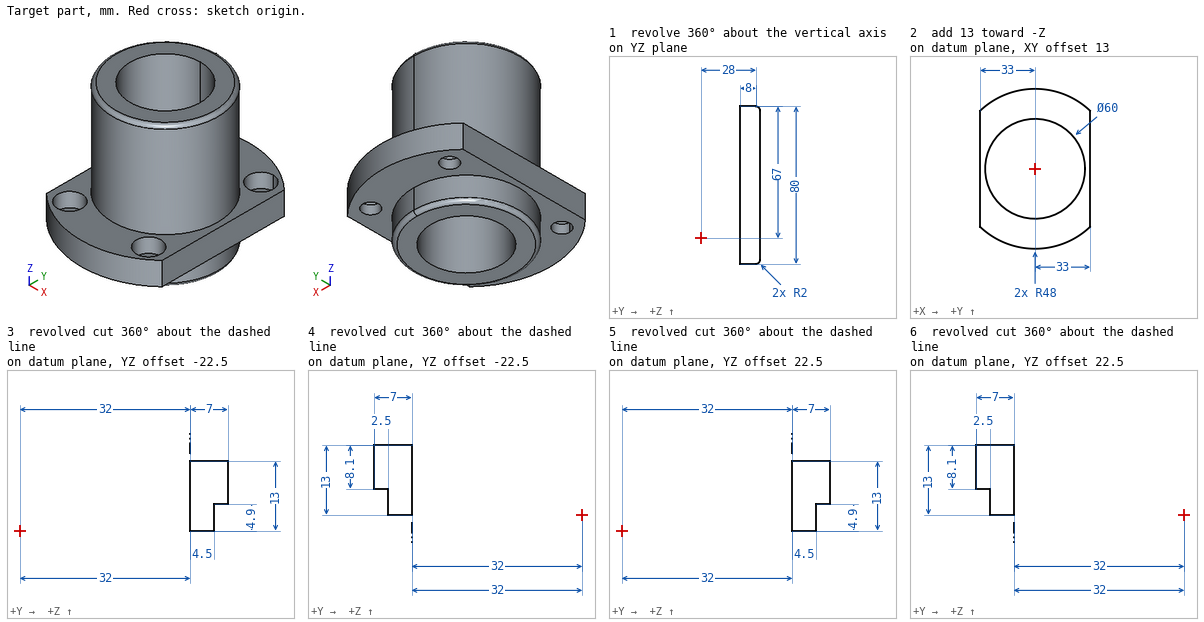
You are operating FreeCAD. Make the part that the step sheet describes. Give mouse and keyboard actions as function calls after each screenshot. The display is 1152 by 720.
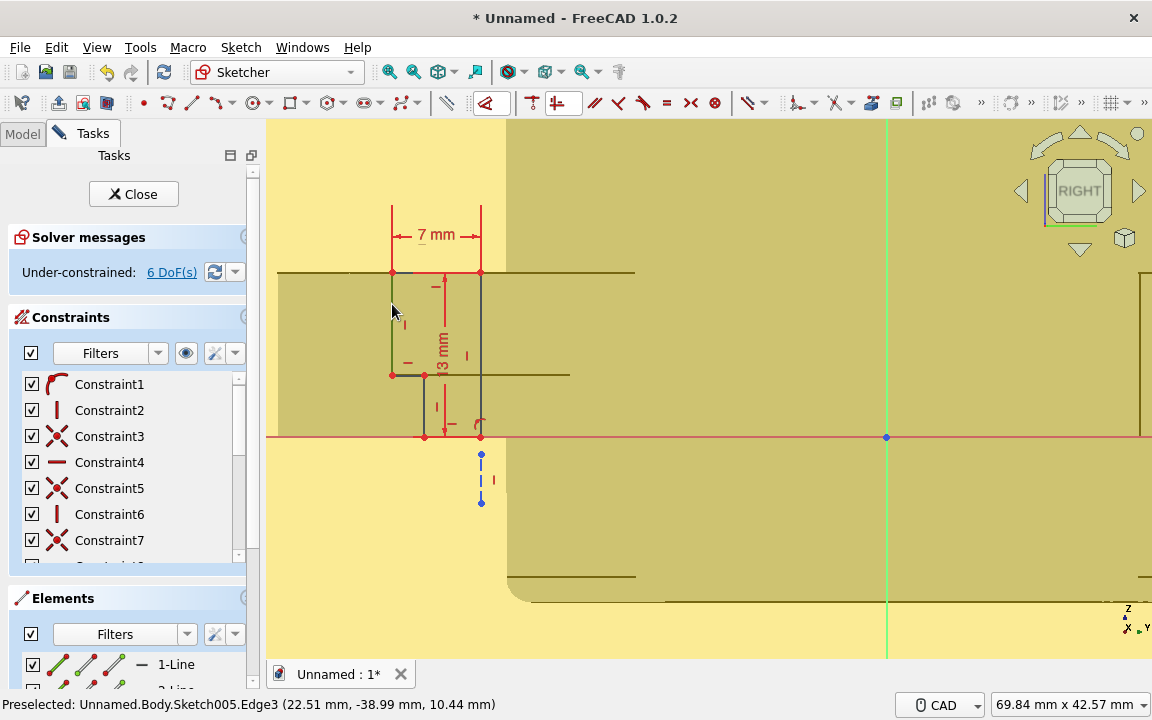
click(504, 104)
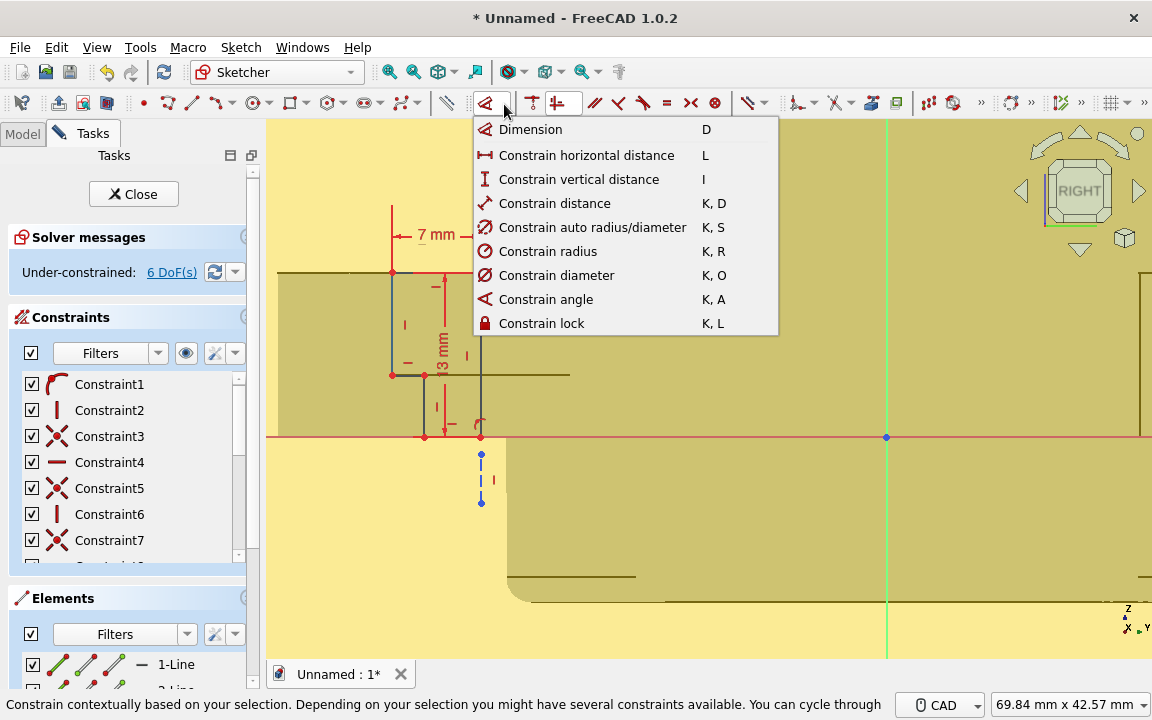
click(626, 179)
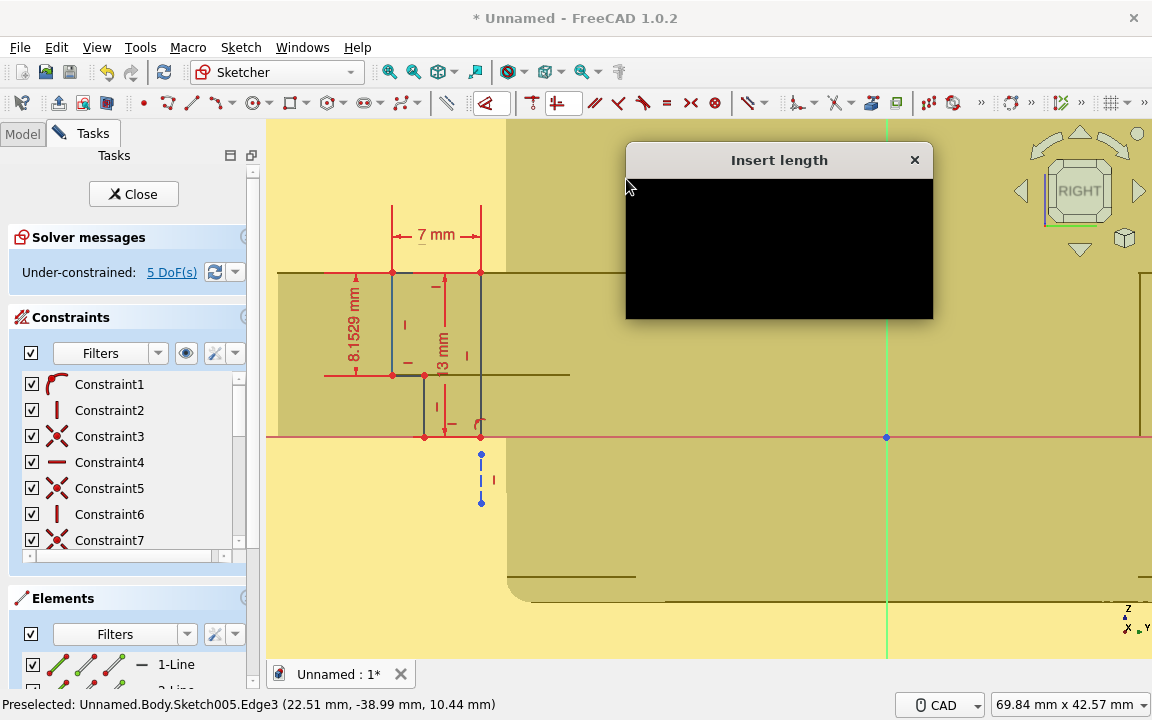
text(8.1)
key(Return)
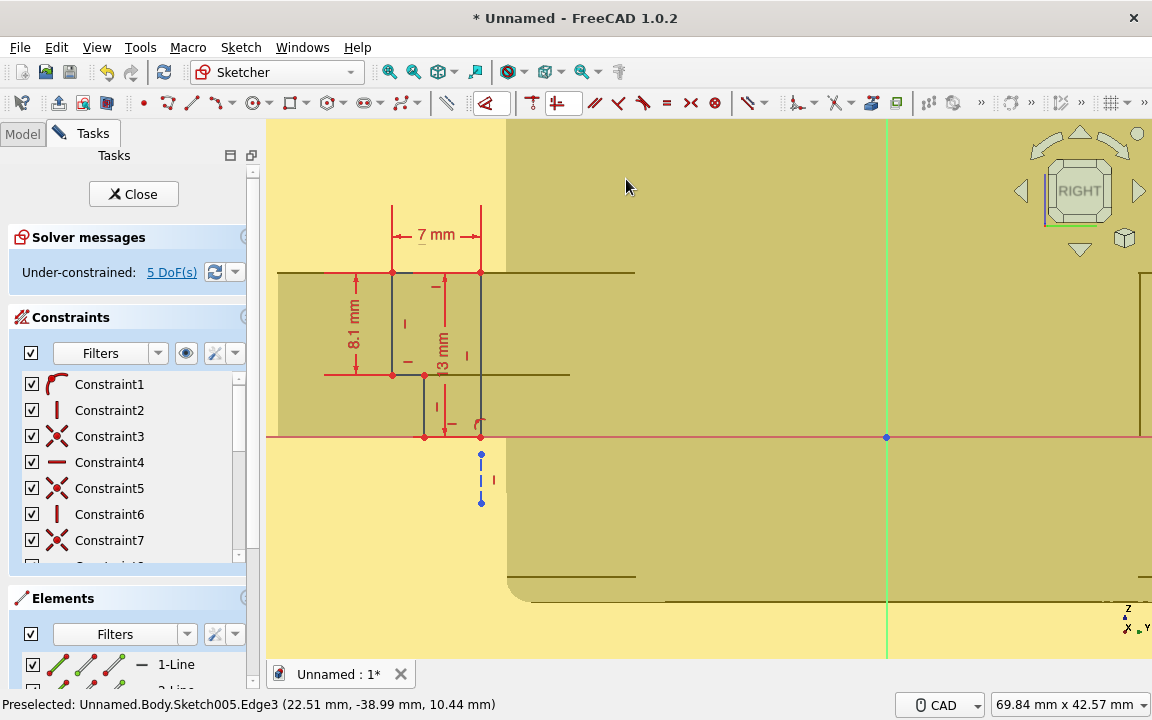
scroll(402, 375, up, 2)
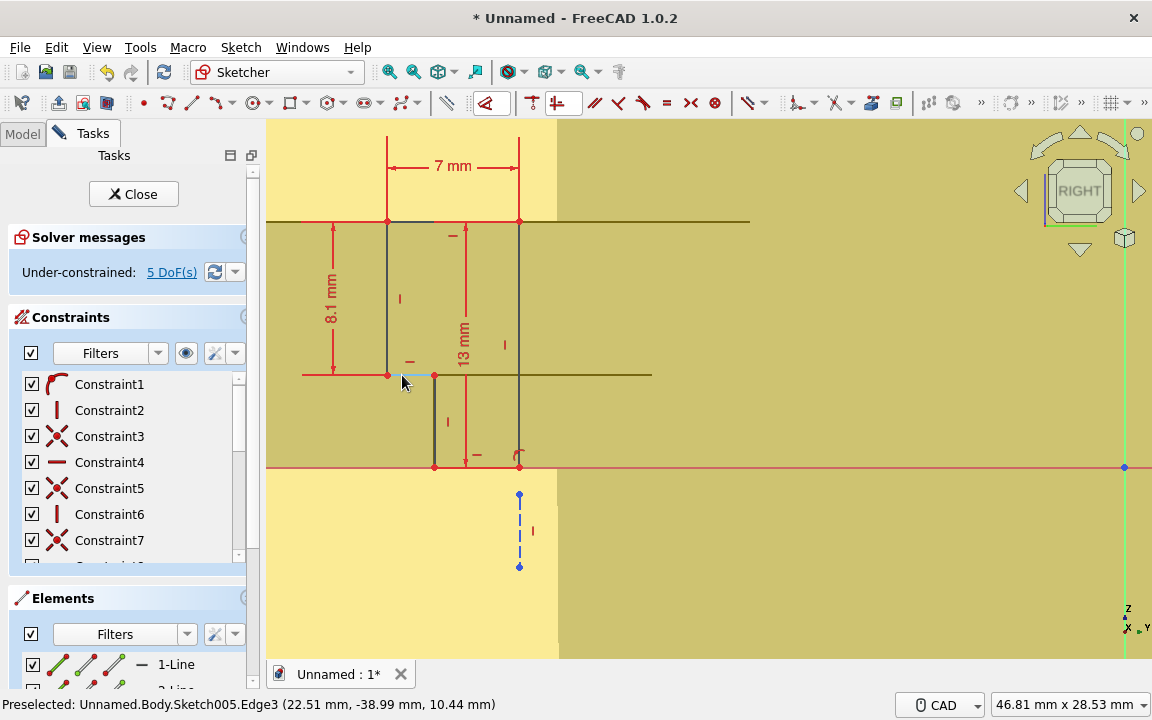
click(401, 375)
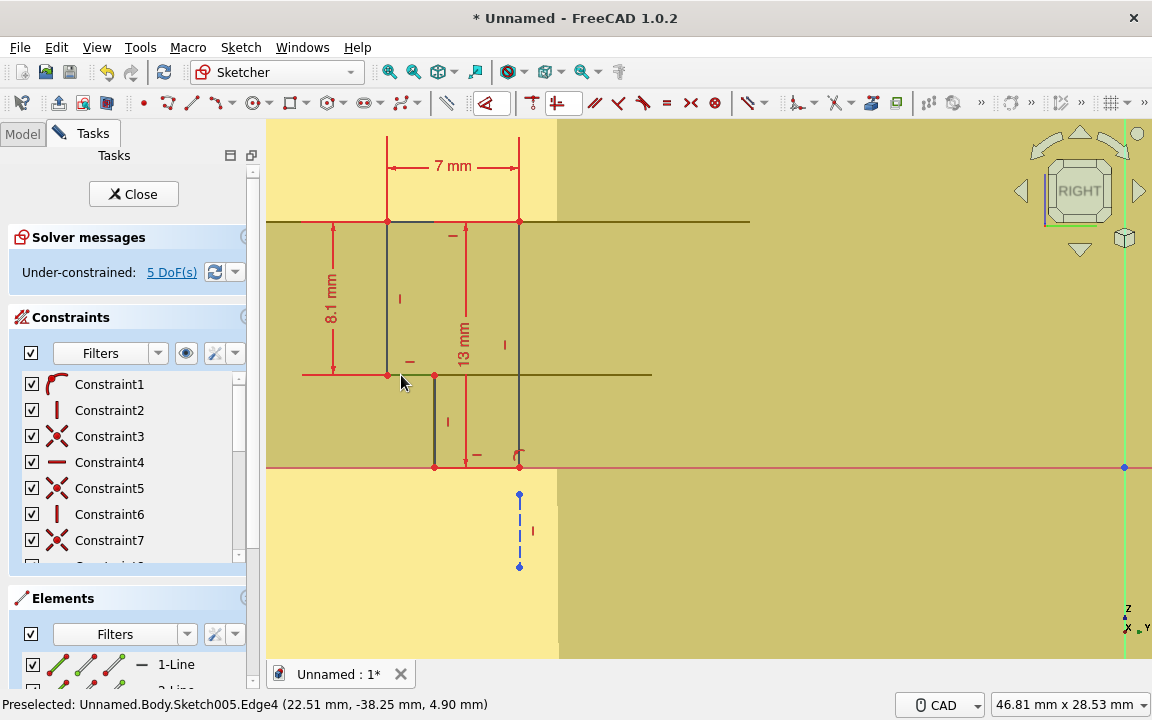
click(504, 104)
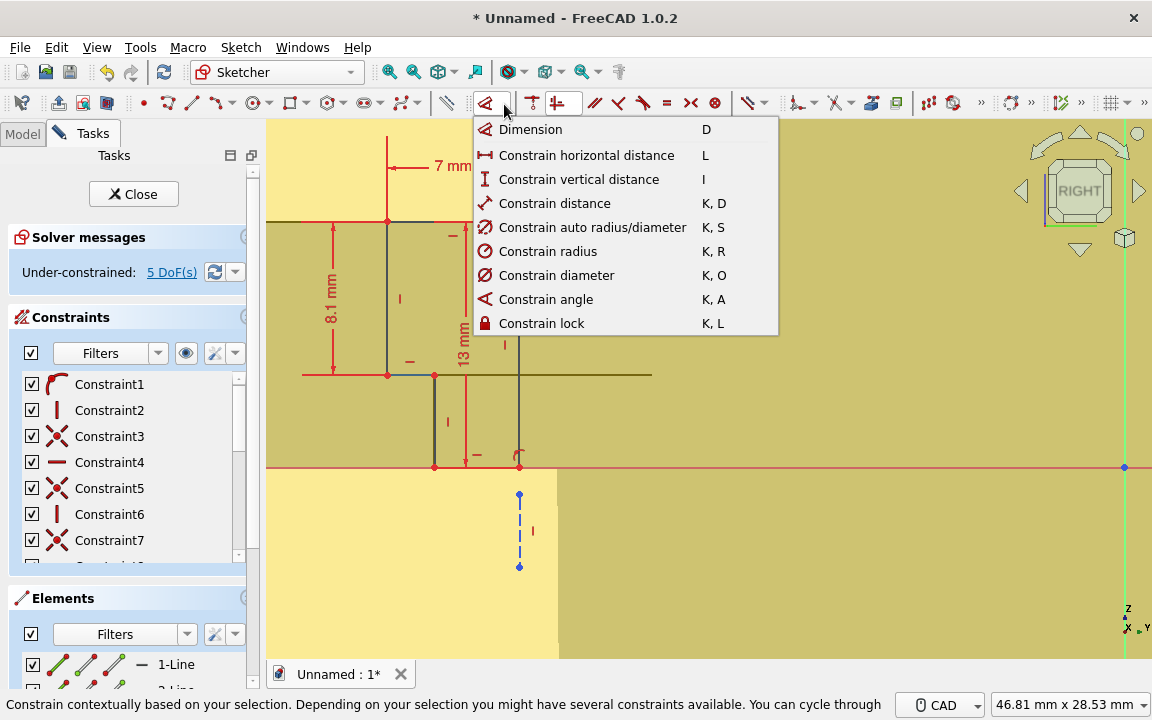
click(626, 155)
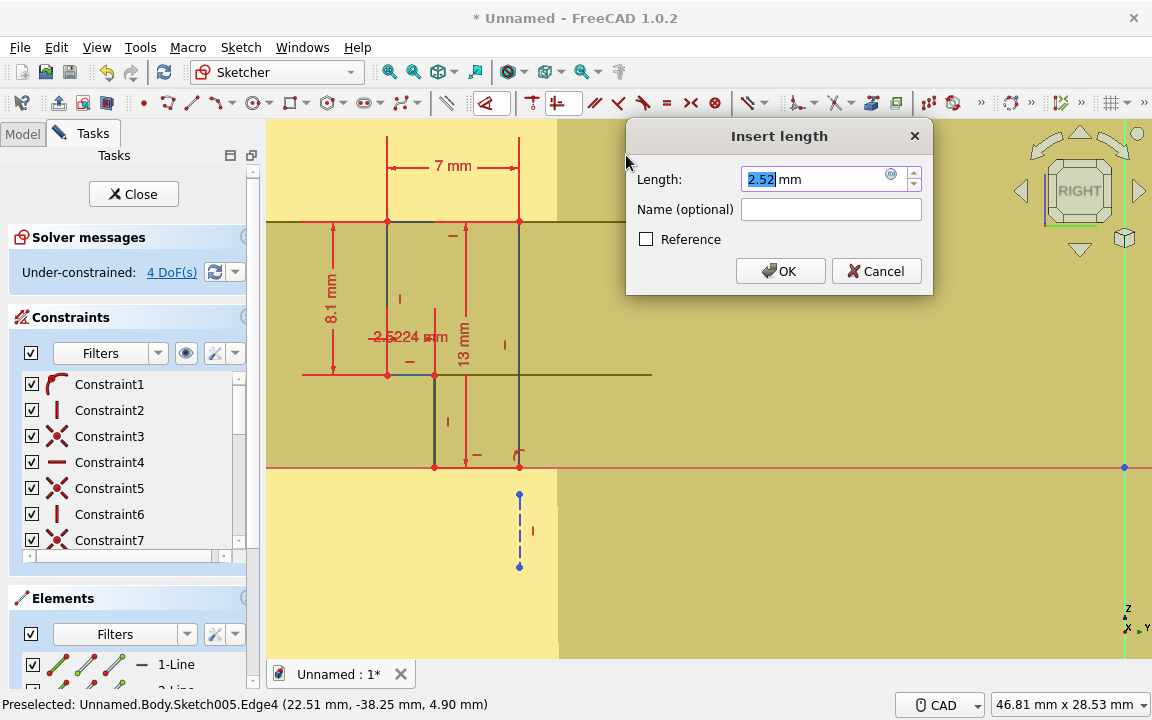
text(2.5)
key(Return)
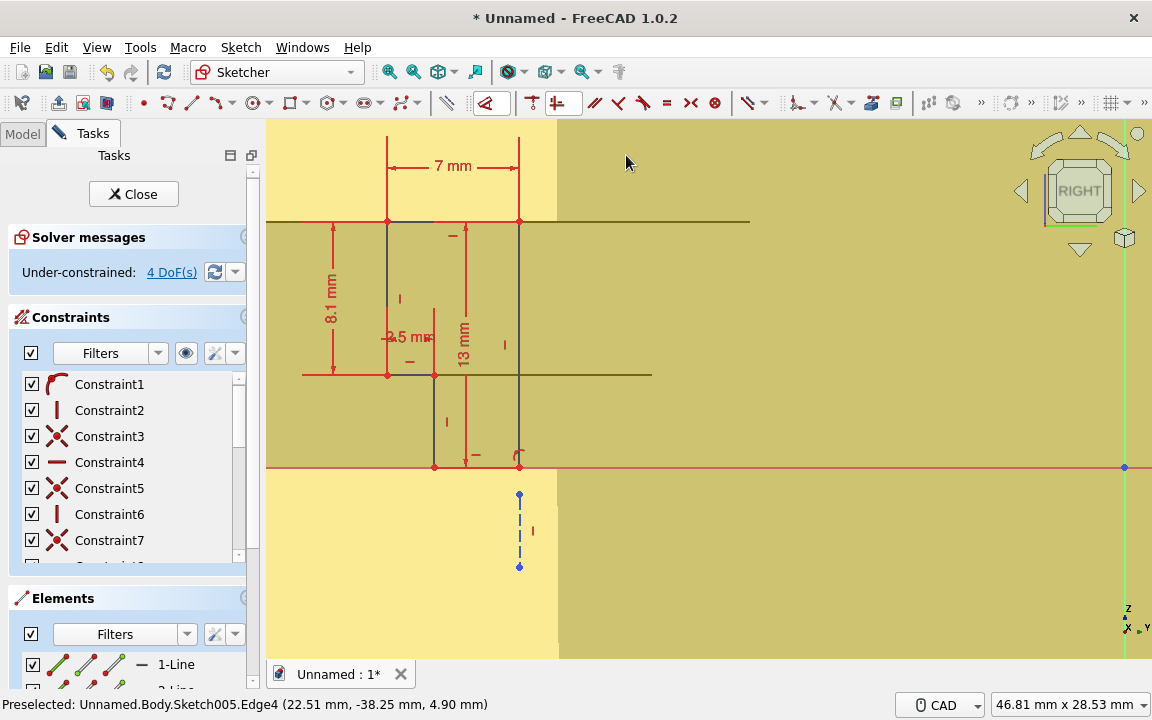
click(519, 468)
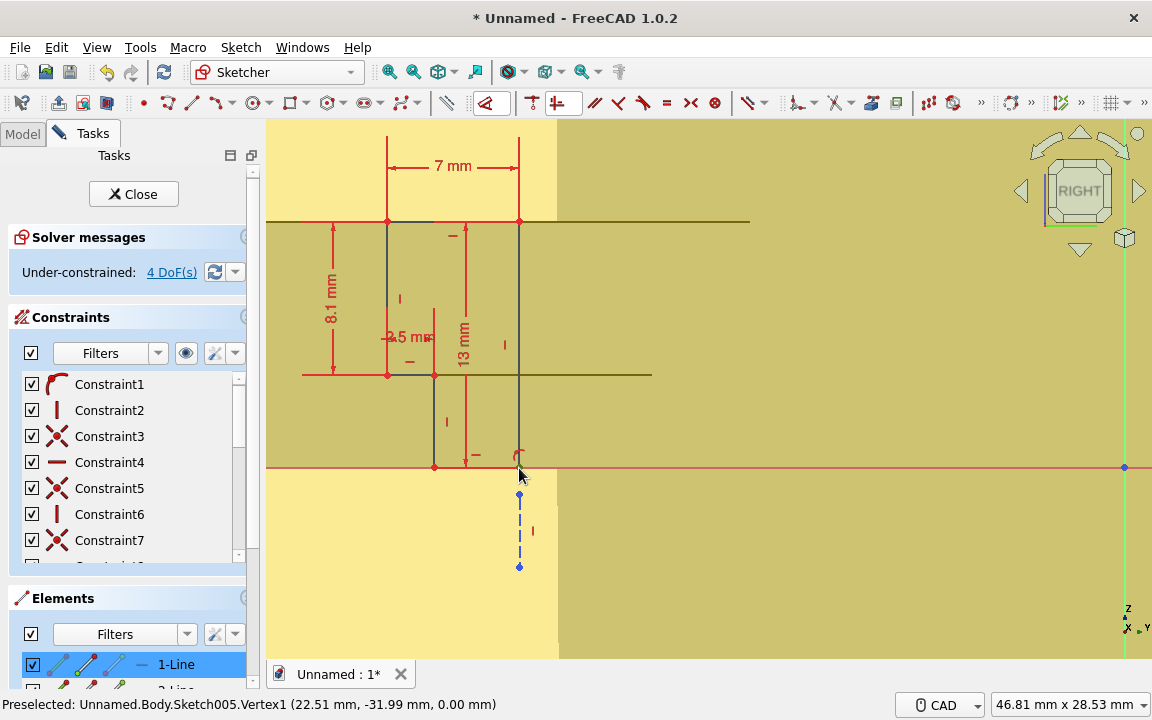
click(504, 104)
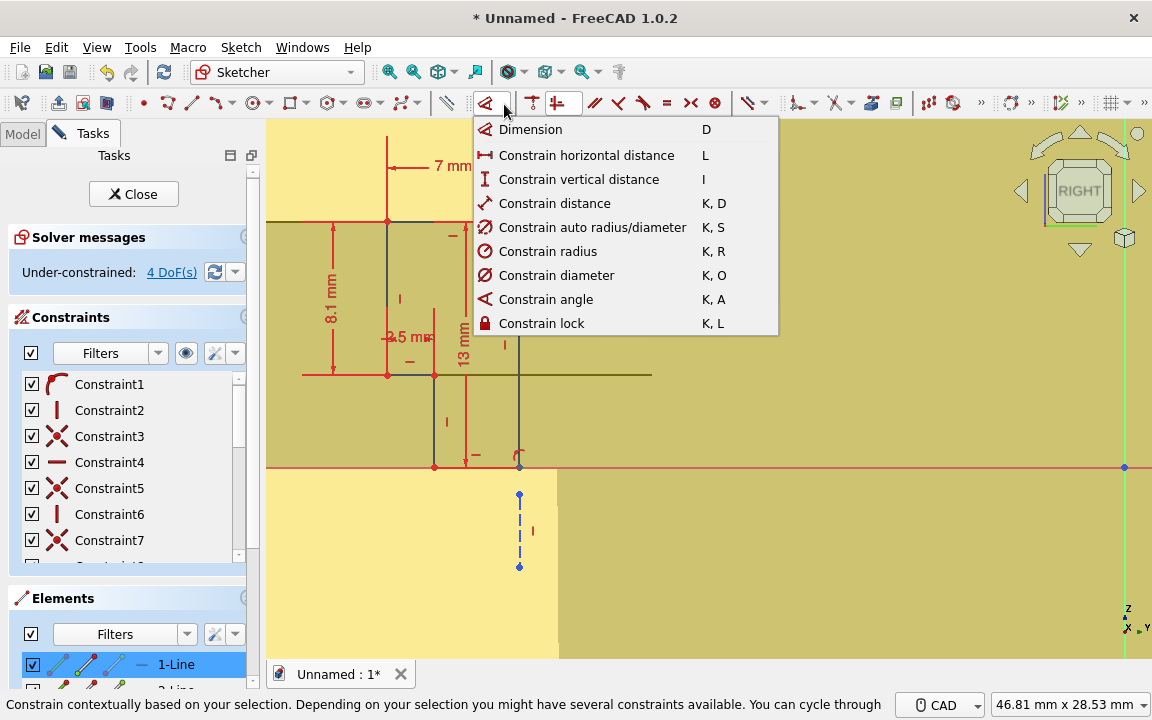
click(626, 155)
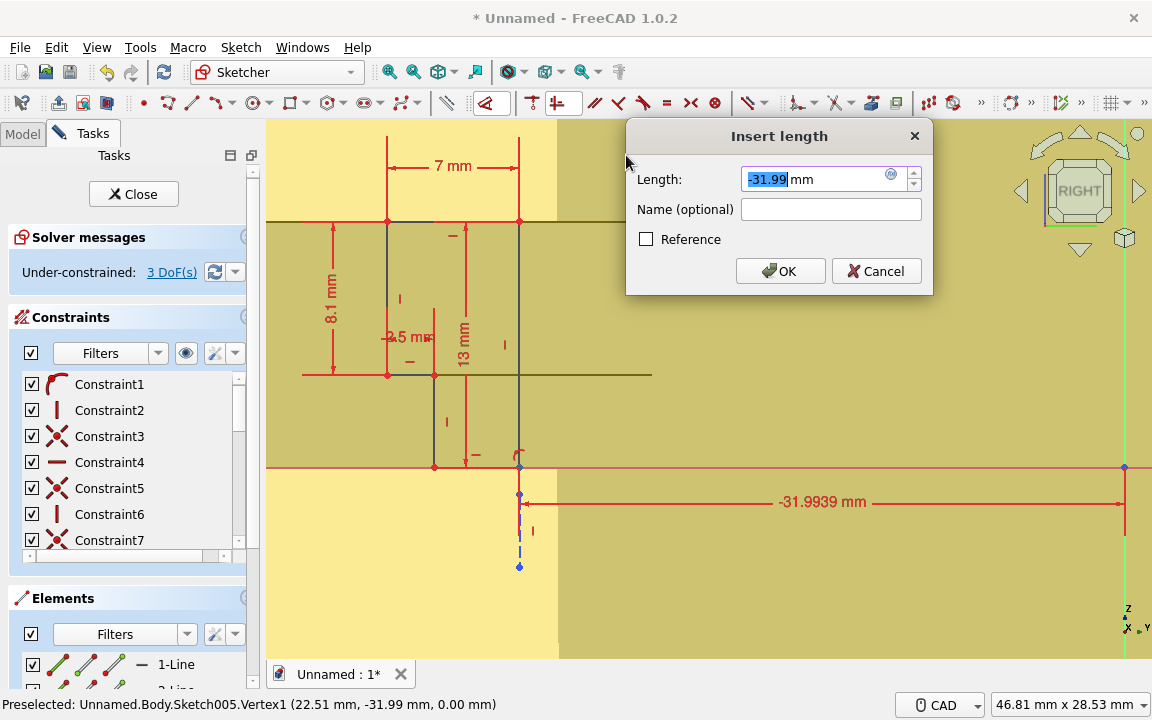
text(-32)
key(Return)